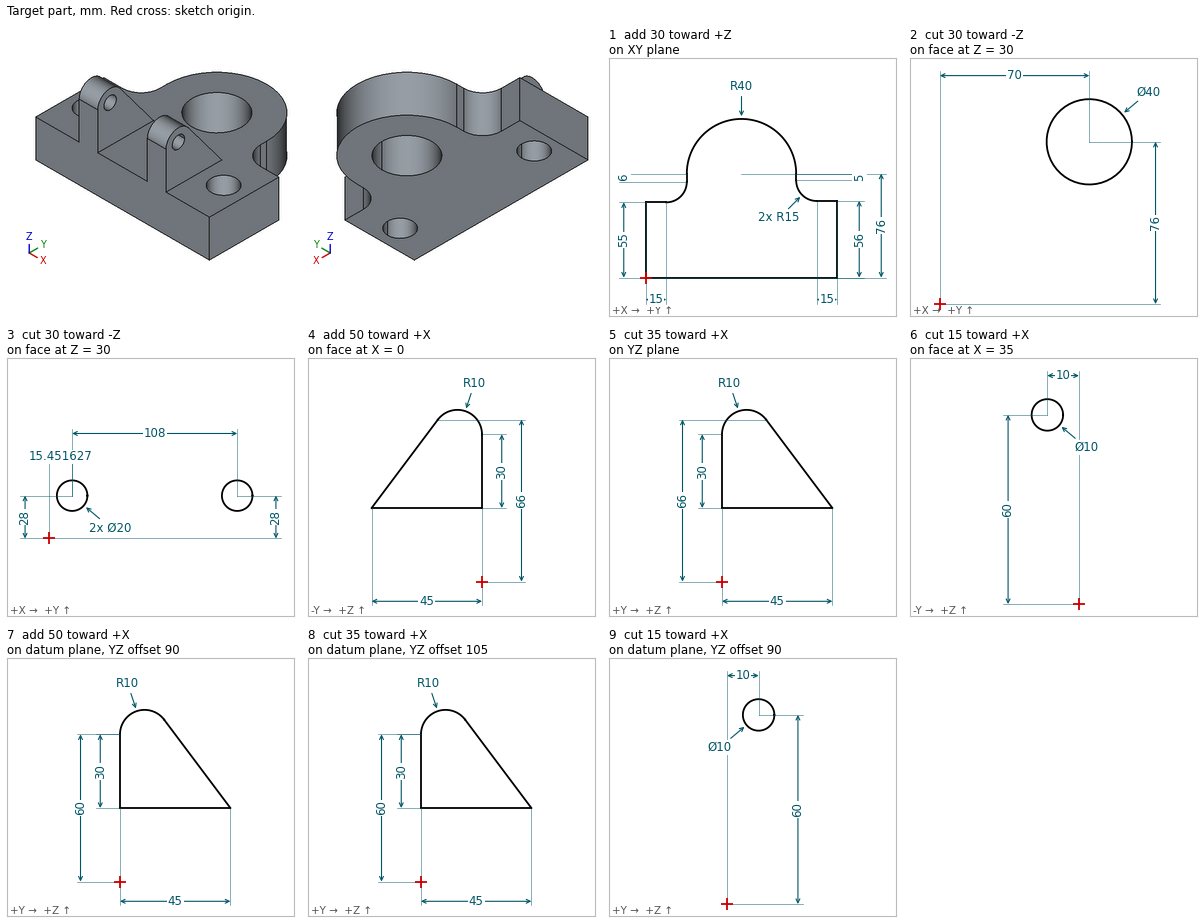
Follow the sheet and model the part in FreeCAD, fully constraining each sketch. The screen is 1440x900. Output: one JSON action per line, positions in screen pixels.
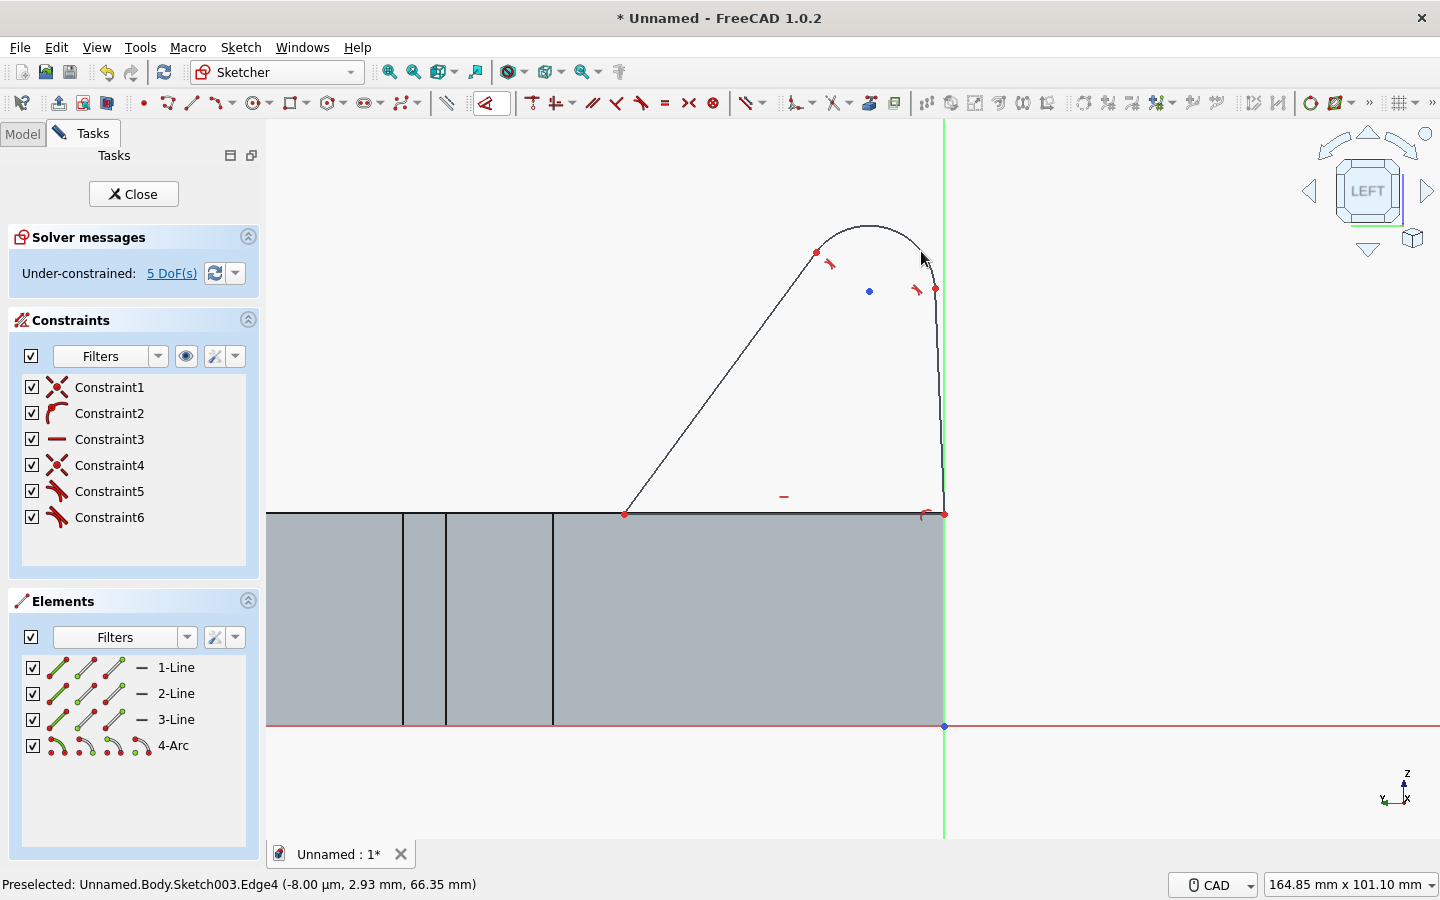
{"action": "left_click", "coordinate": [942, 447]}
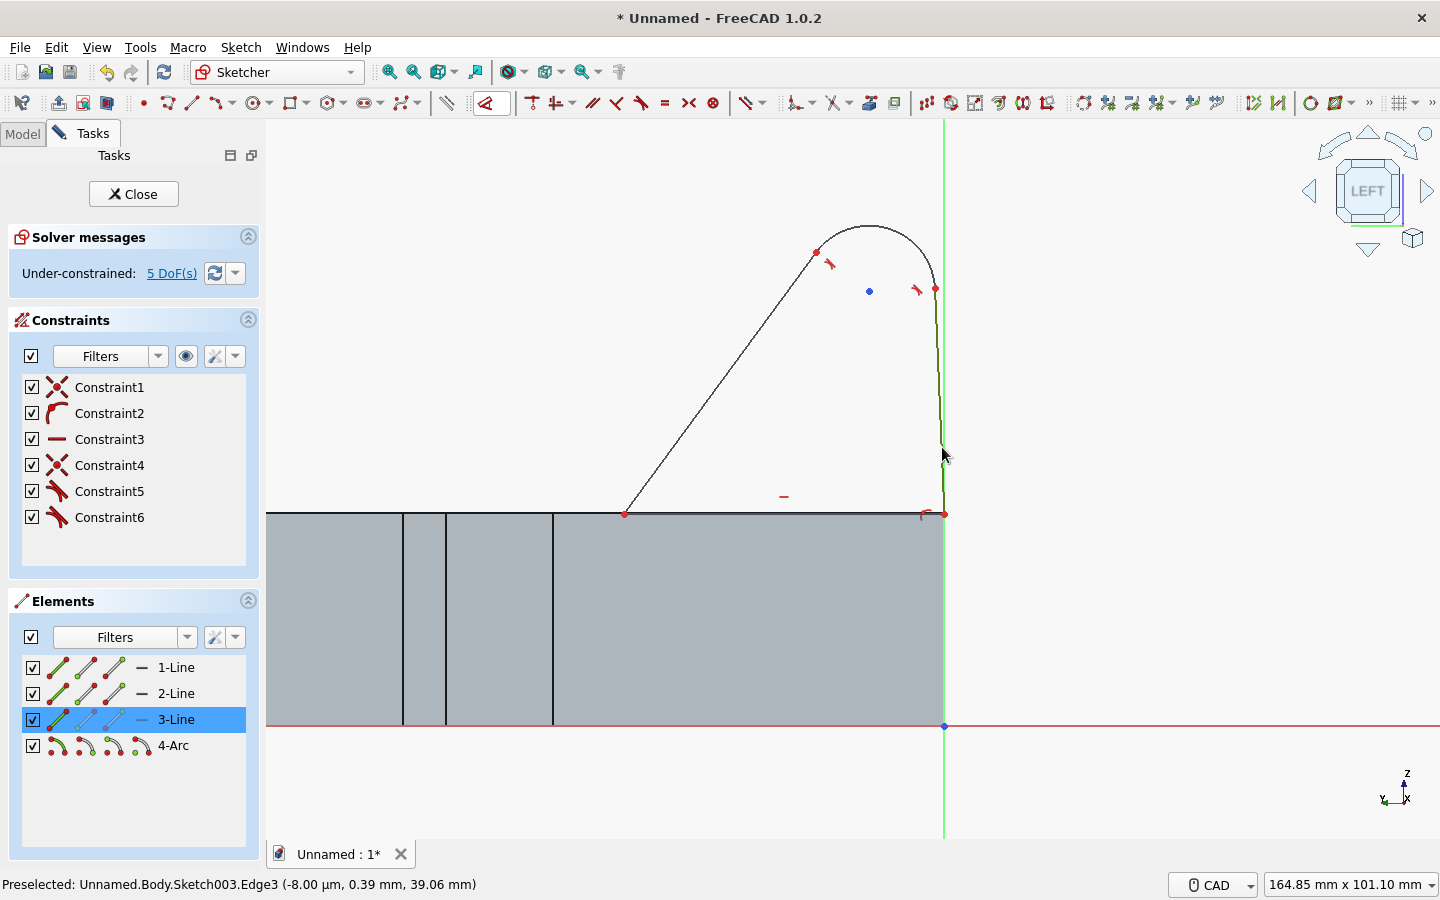
{"action": "key", "text": "v"}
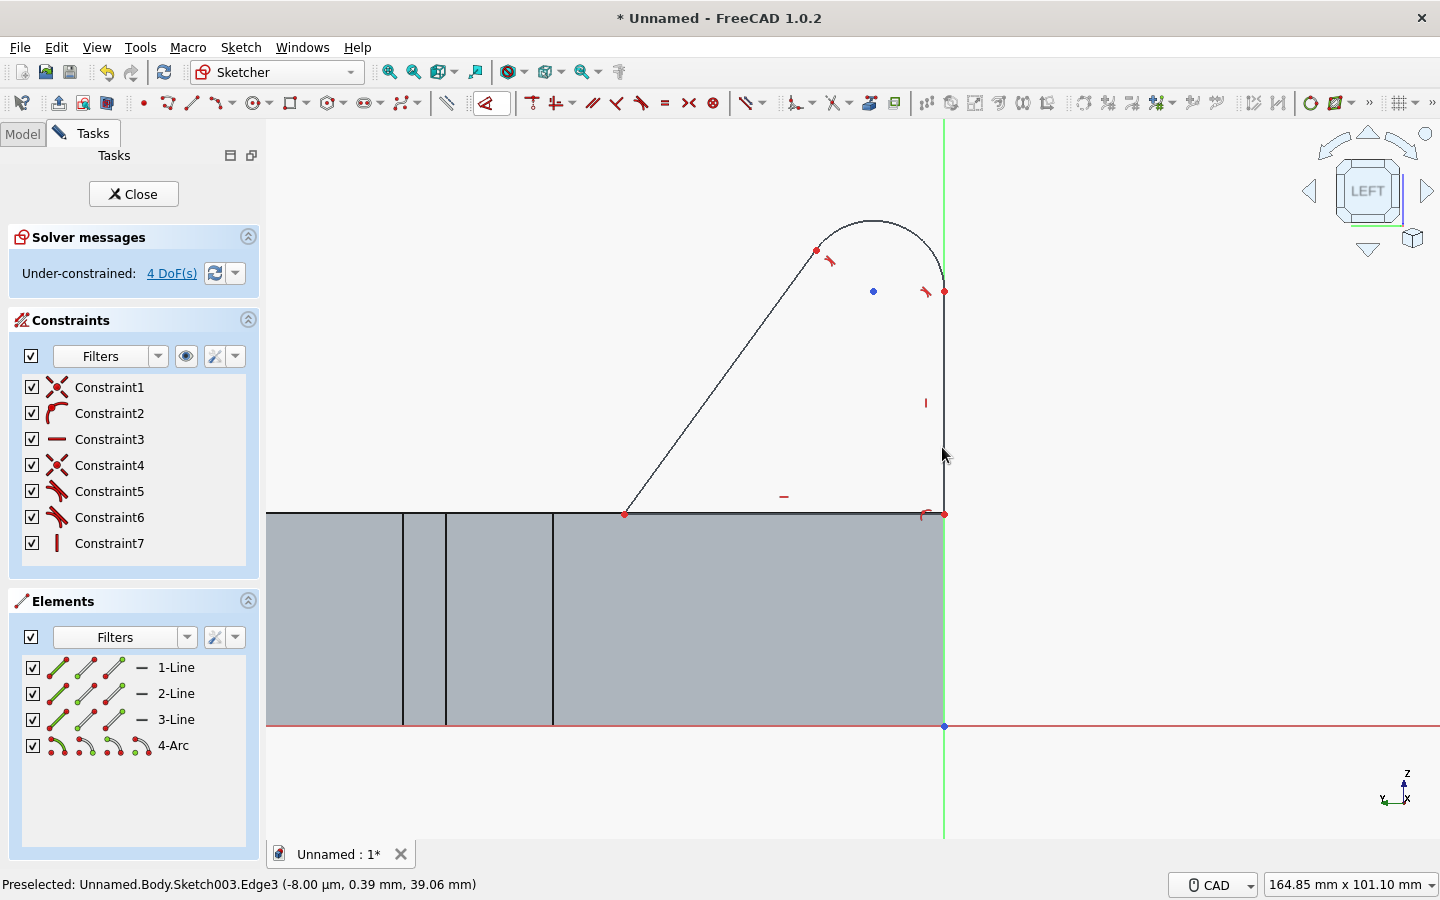
{"action": "left_click", "coordinate": [925, 243]}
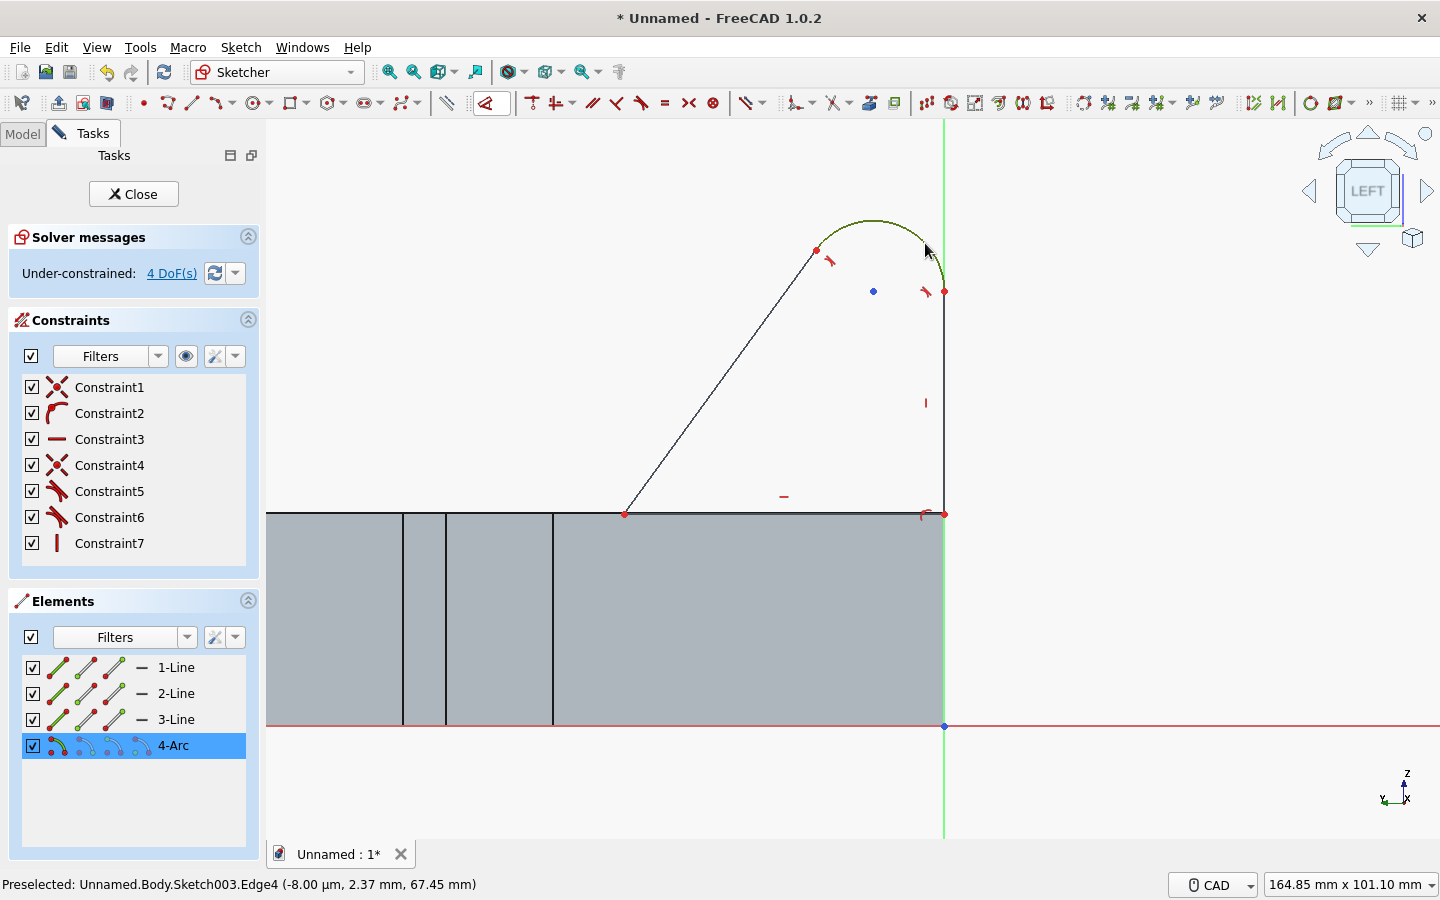
{"action": "key", "text": "k r"}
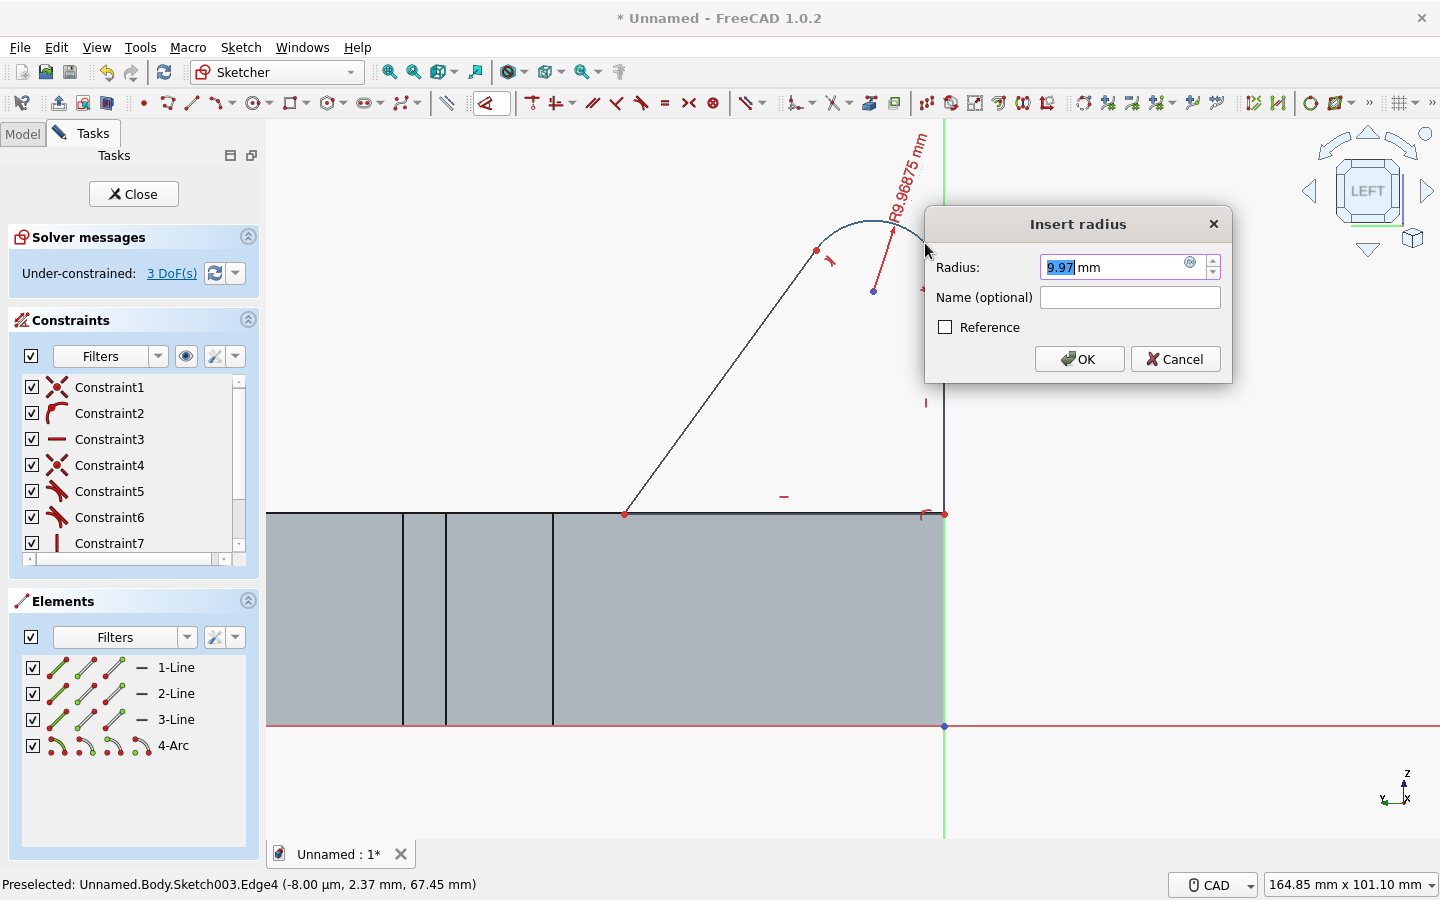
{"action": "type", "text": "10"}
{"action": "key", "text": "Return"}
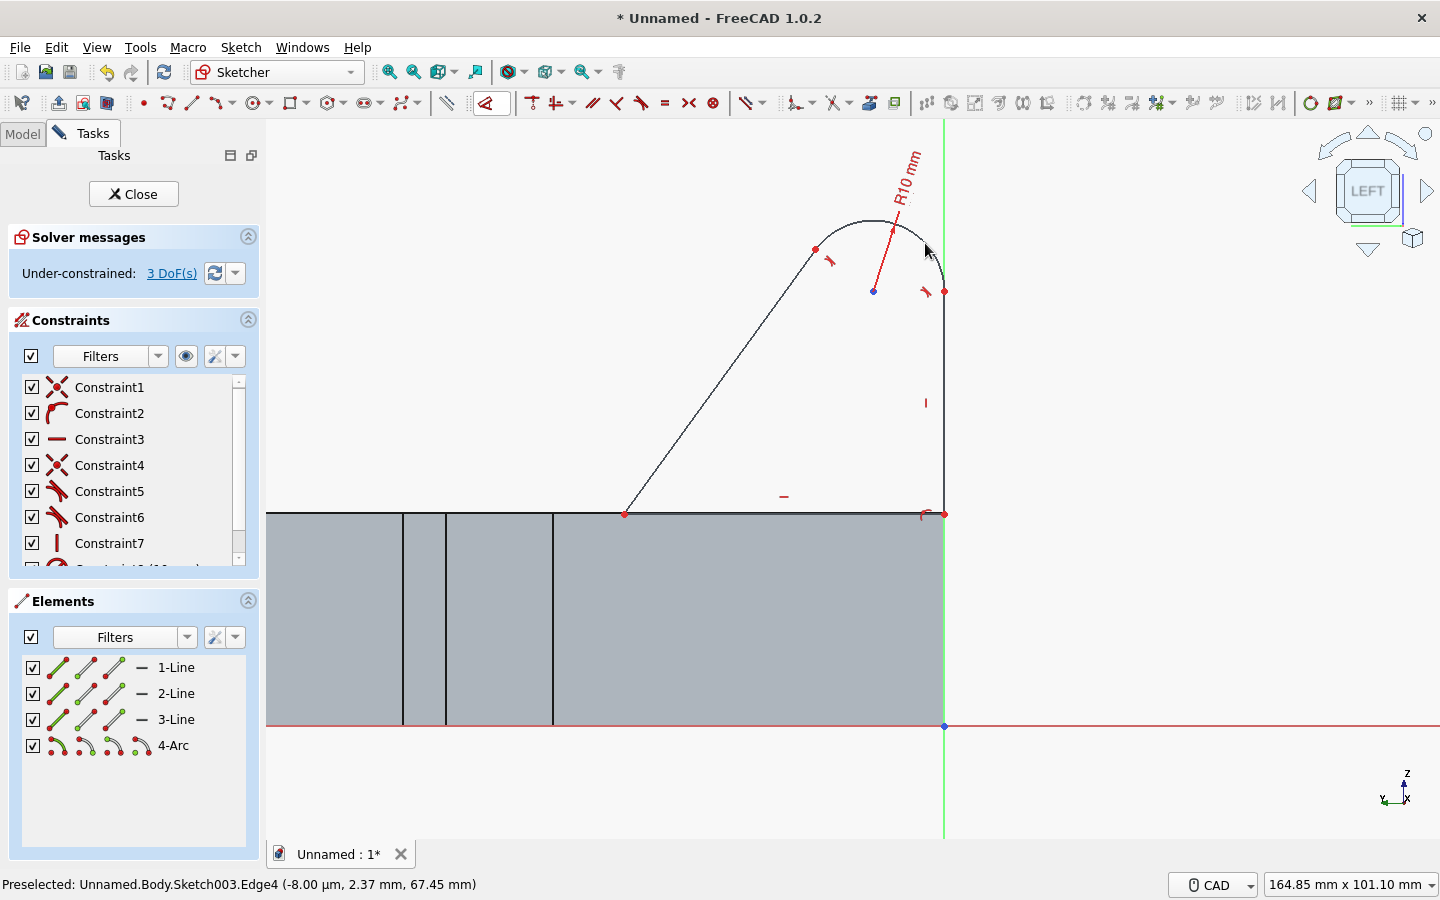
{"action": "left_click", "coordinate": [720, 514]}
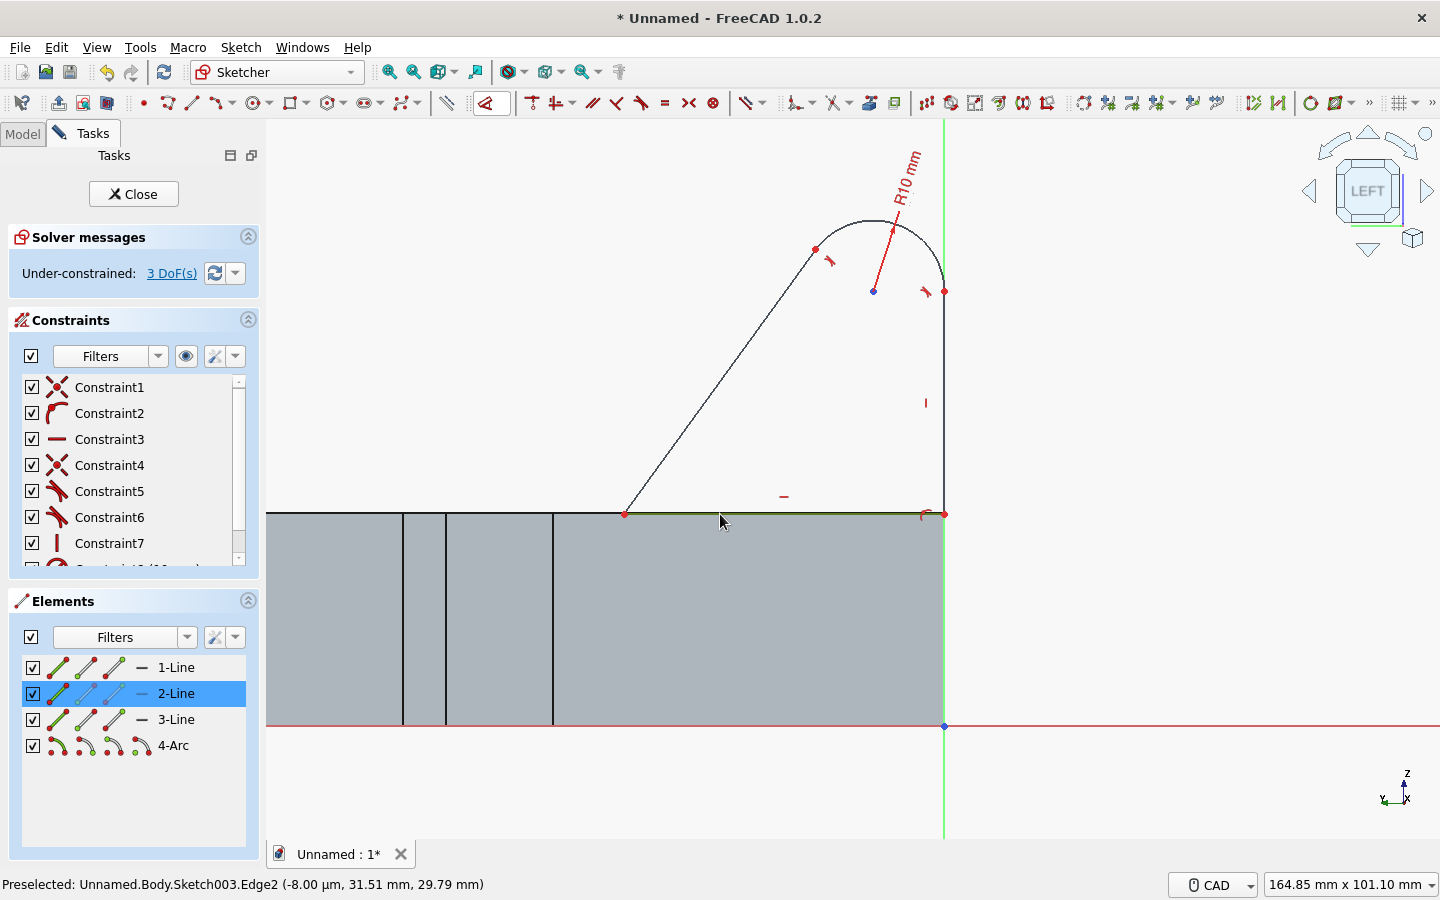
{"action": "left_click", "coordinate": [504, 104]}